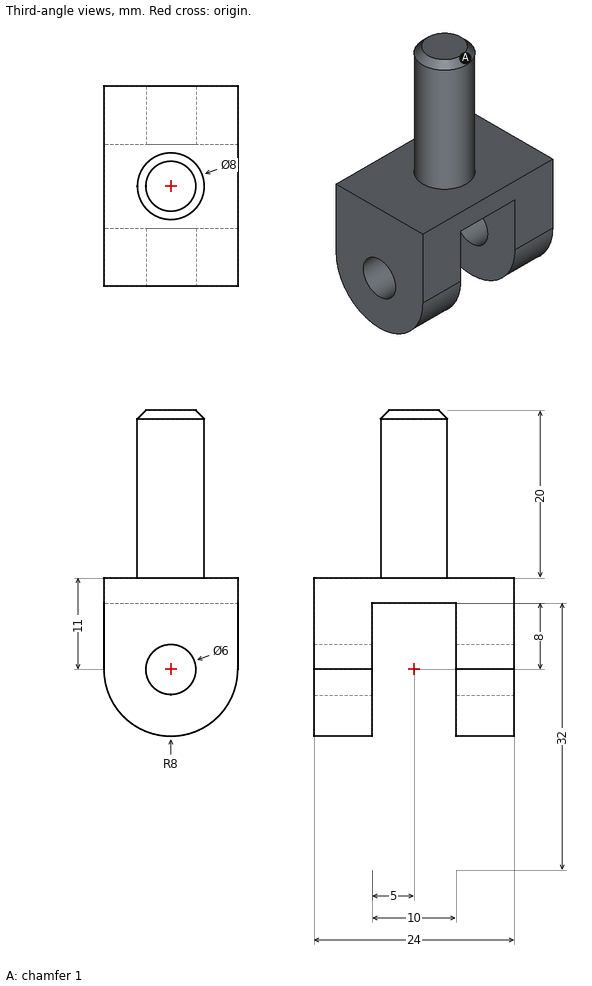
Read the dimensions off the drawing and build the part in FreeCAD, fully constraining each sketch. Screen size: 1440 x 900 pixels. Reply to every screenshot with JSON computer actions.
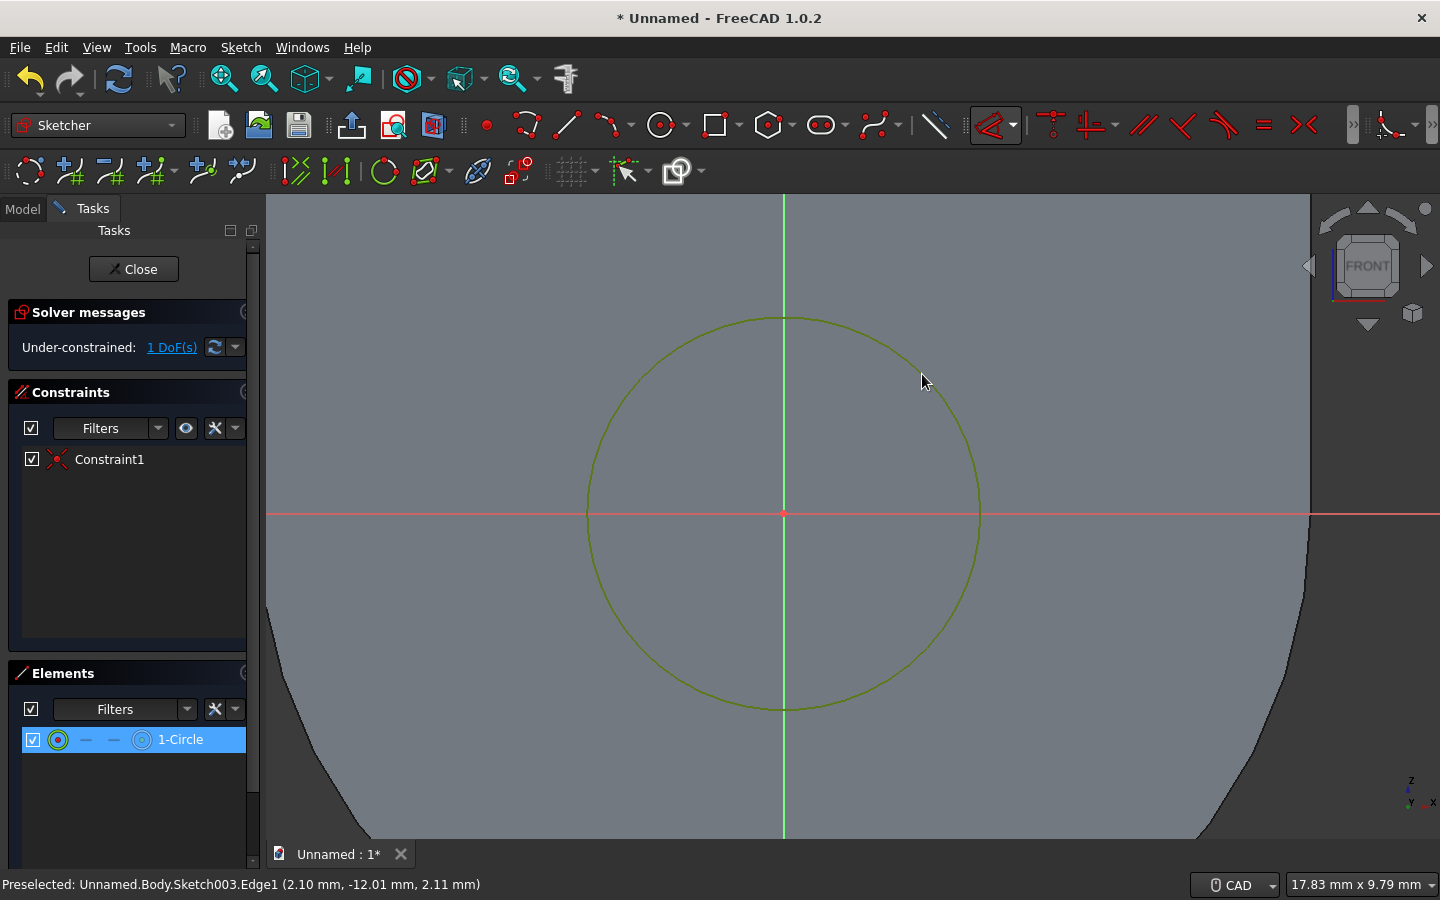
{"action": "left_click", "coordinate": [1016, 126]}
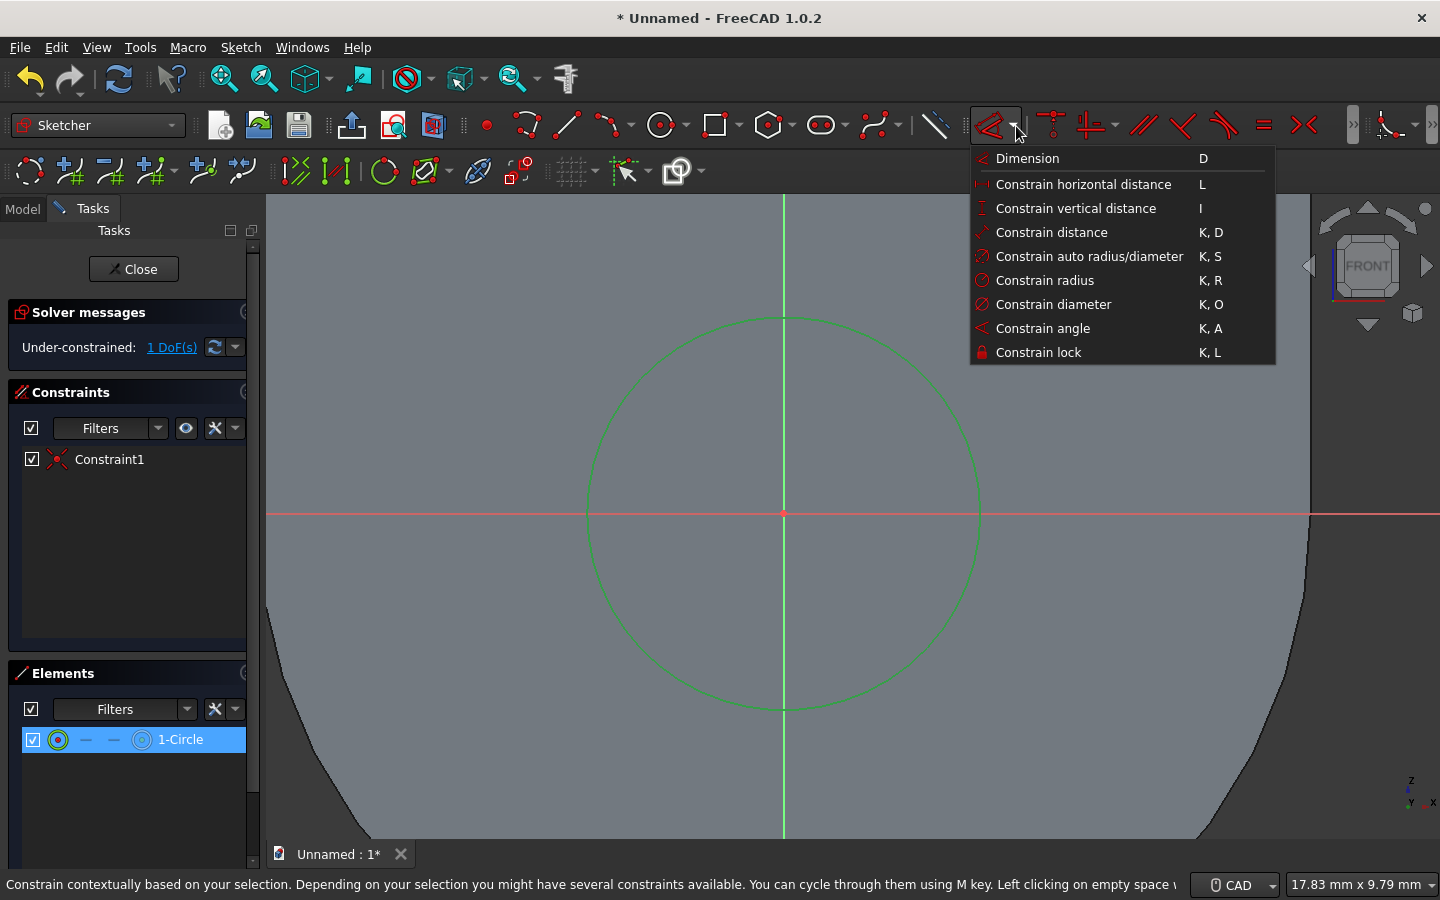
{"action": "left_click", "coordinate": [1123, 304]}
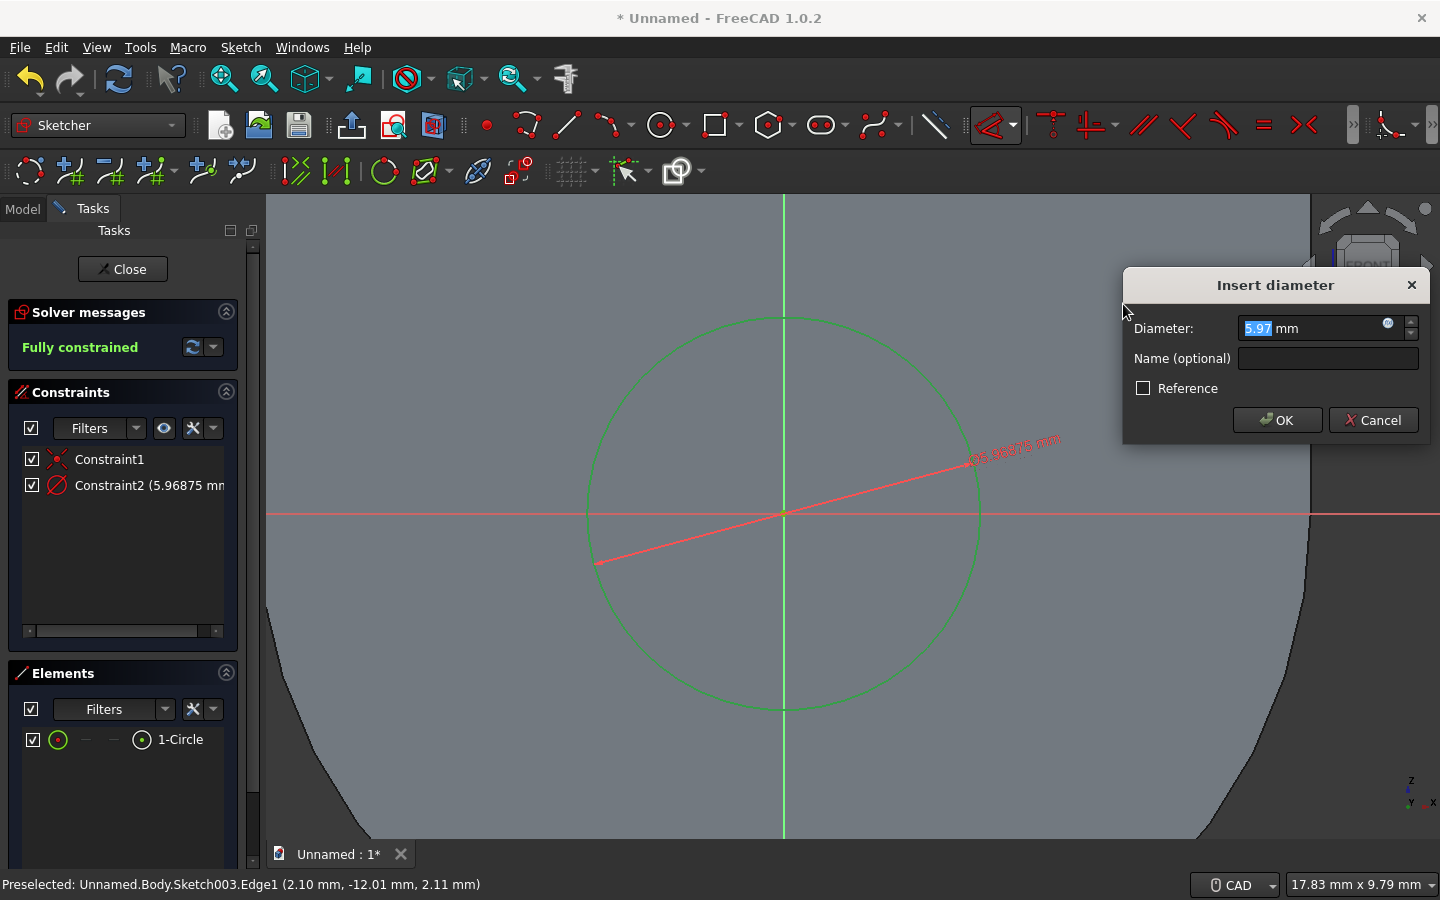
{"action": "type", "text": "6"}
{"action": "key", "text": "Return"}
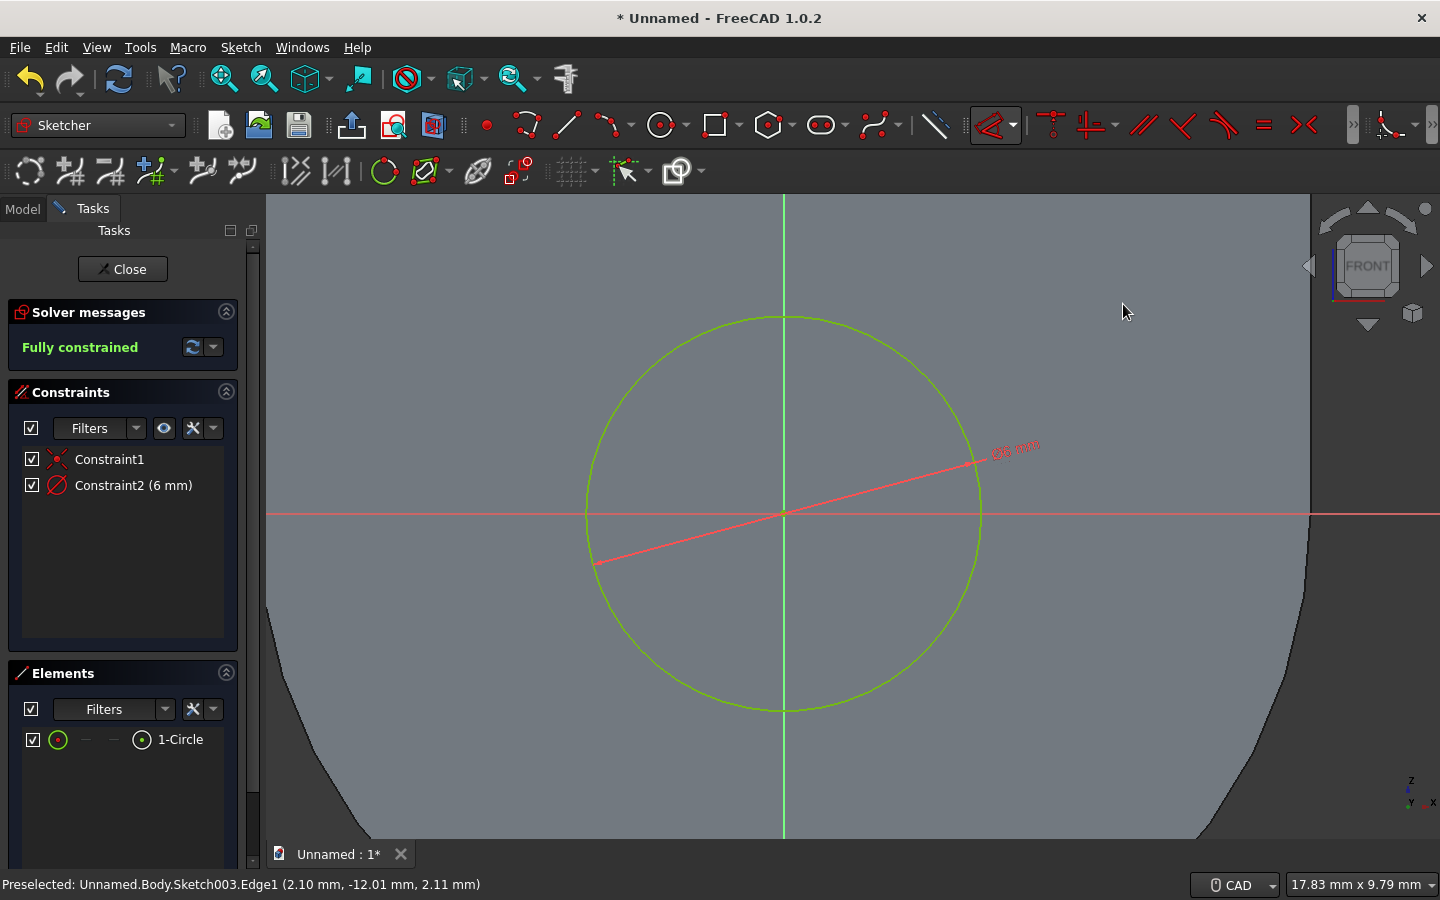
{"action": "left_click", "coordinate": [123, 269]}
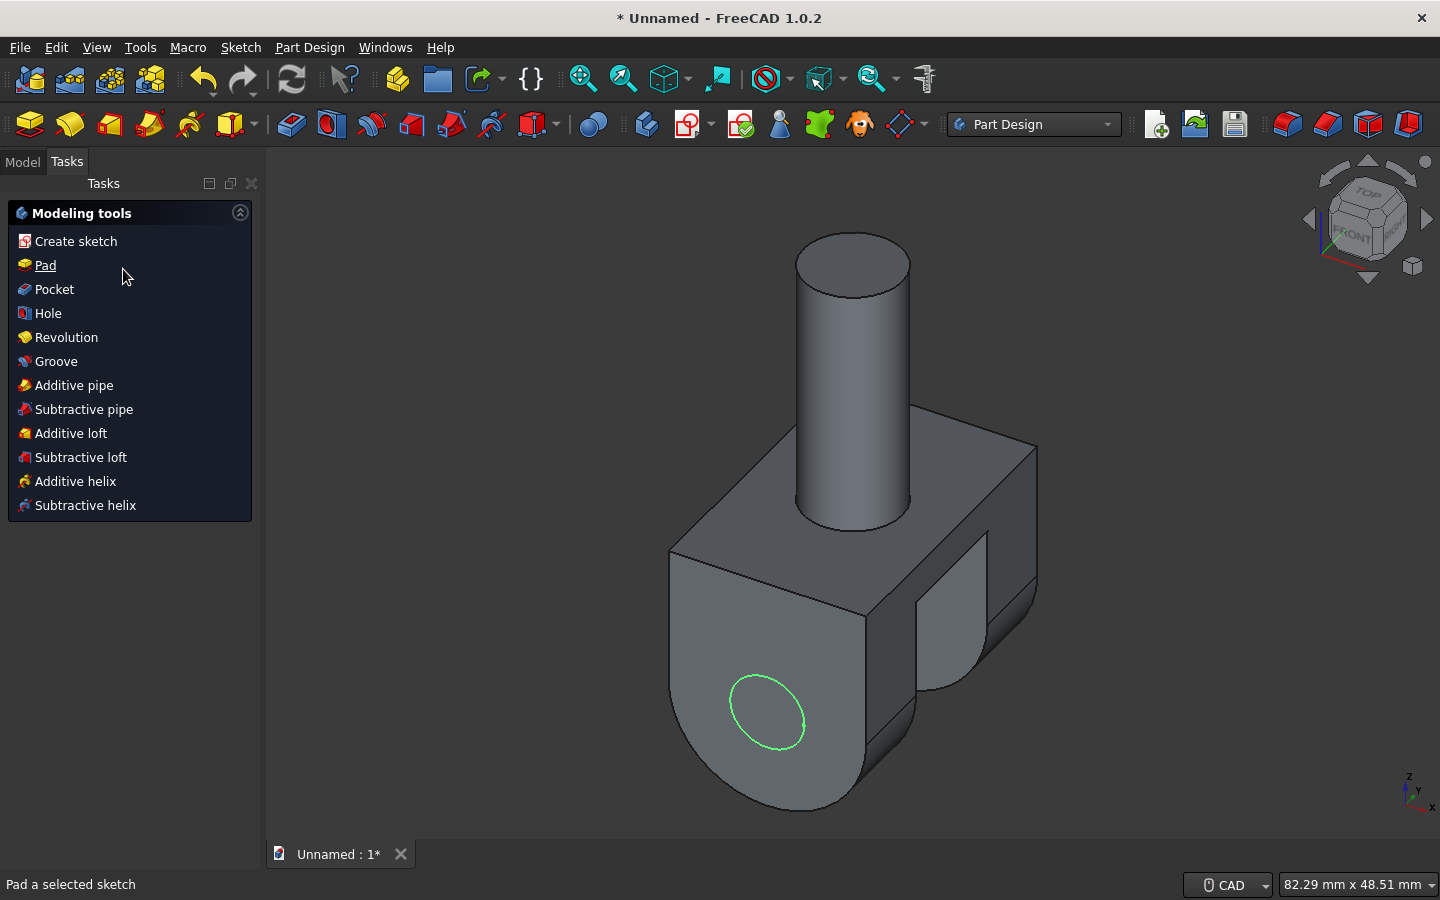
{"action": "left_click", "coordinate": [292, 124]}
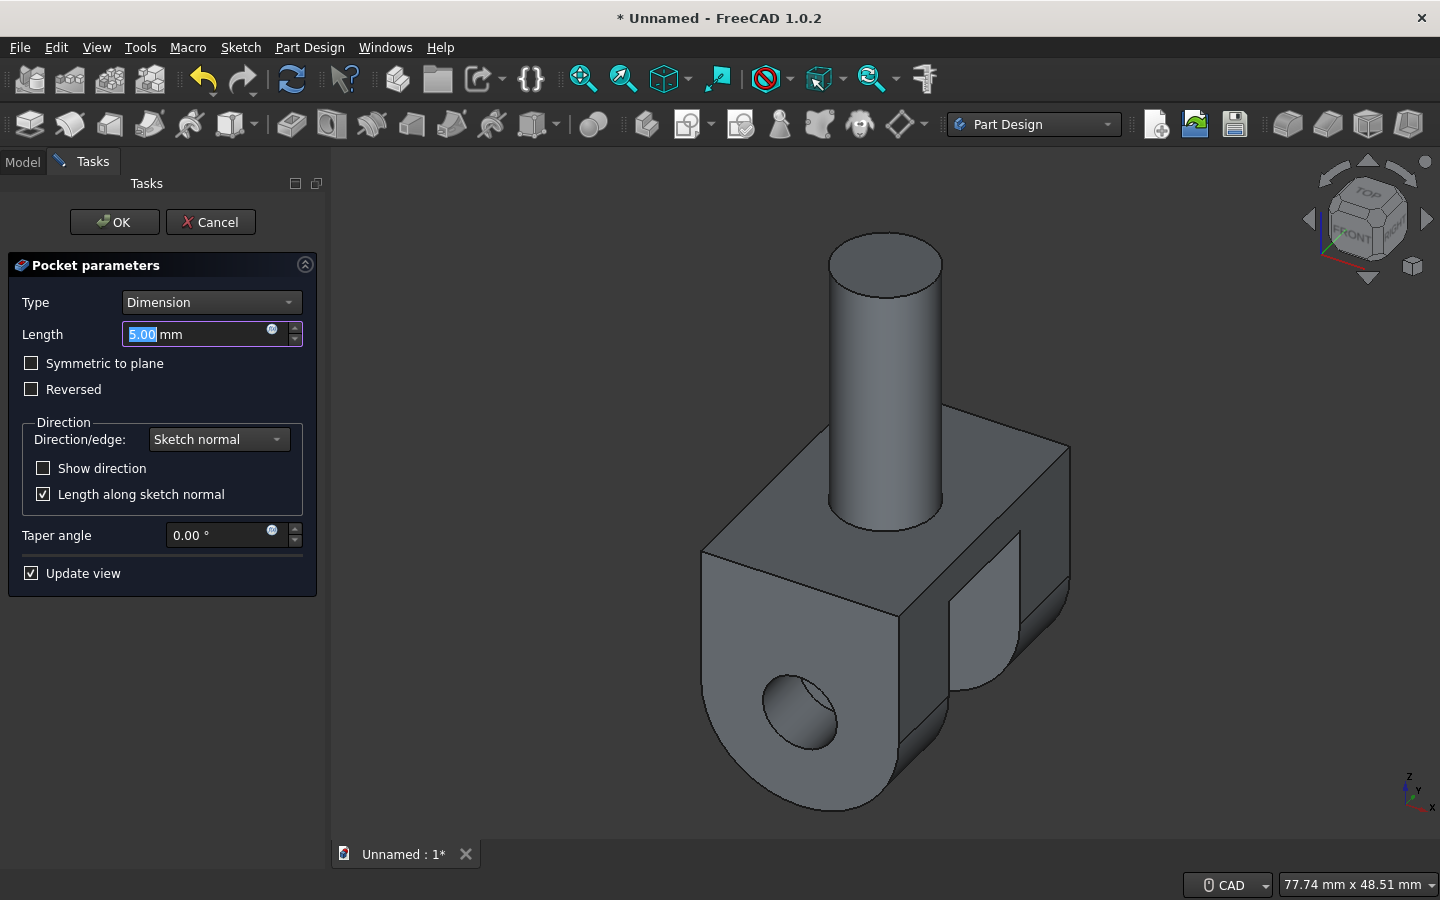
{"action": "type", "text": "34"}
{"action": "key", "text": "Tab"}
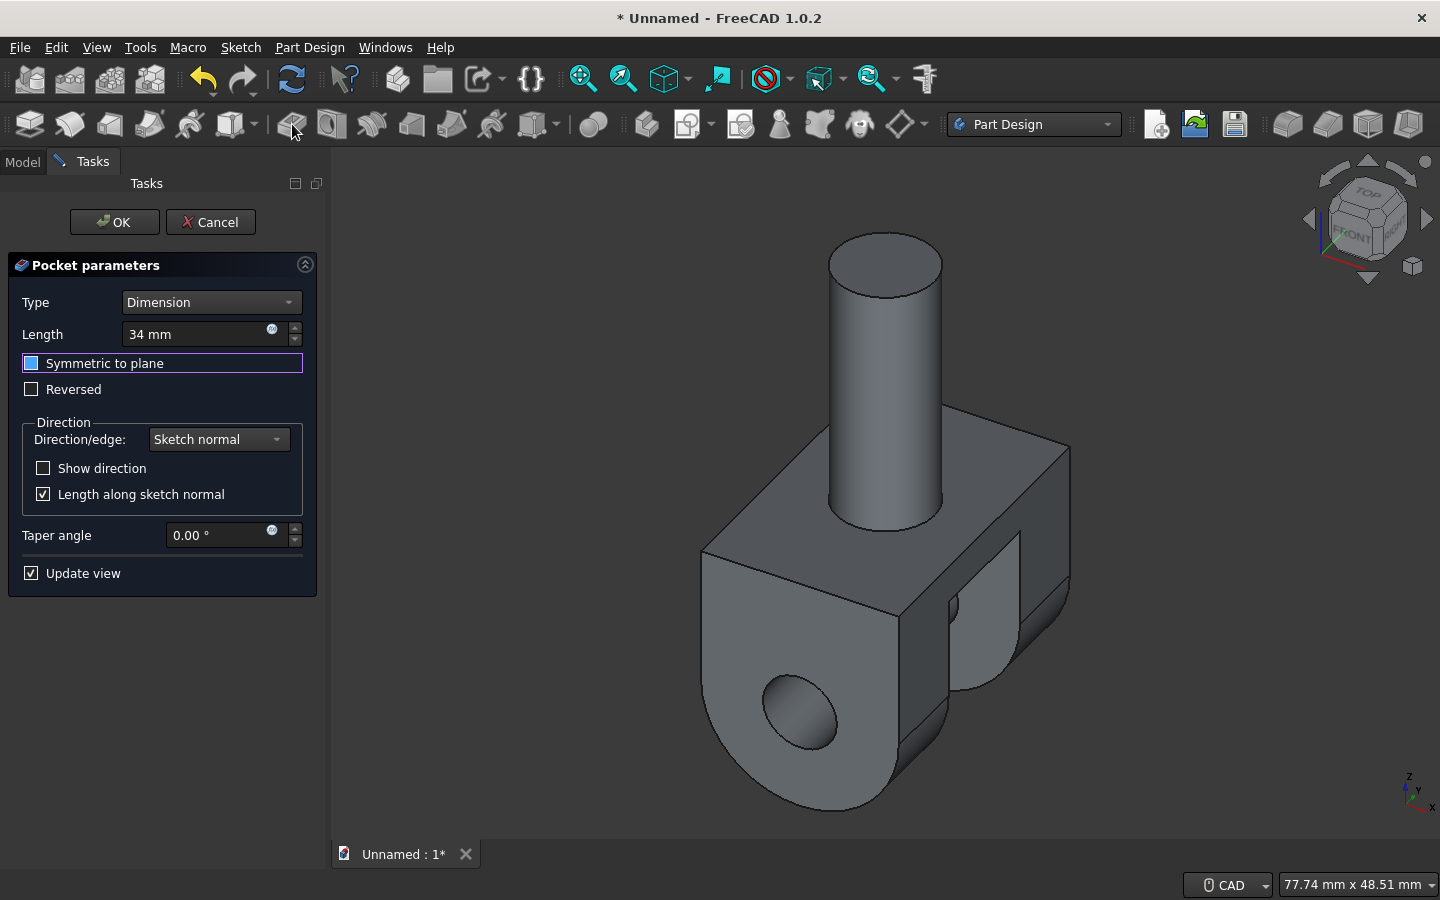
{"action": "left_click", "coordinate": [115, 222]}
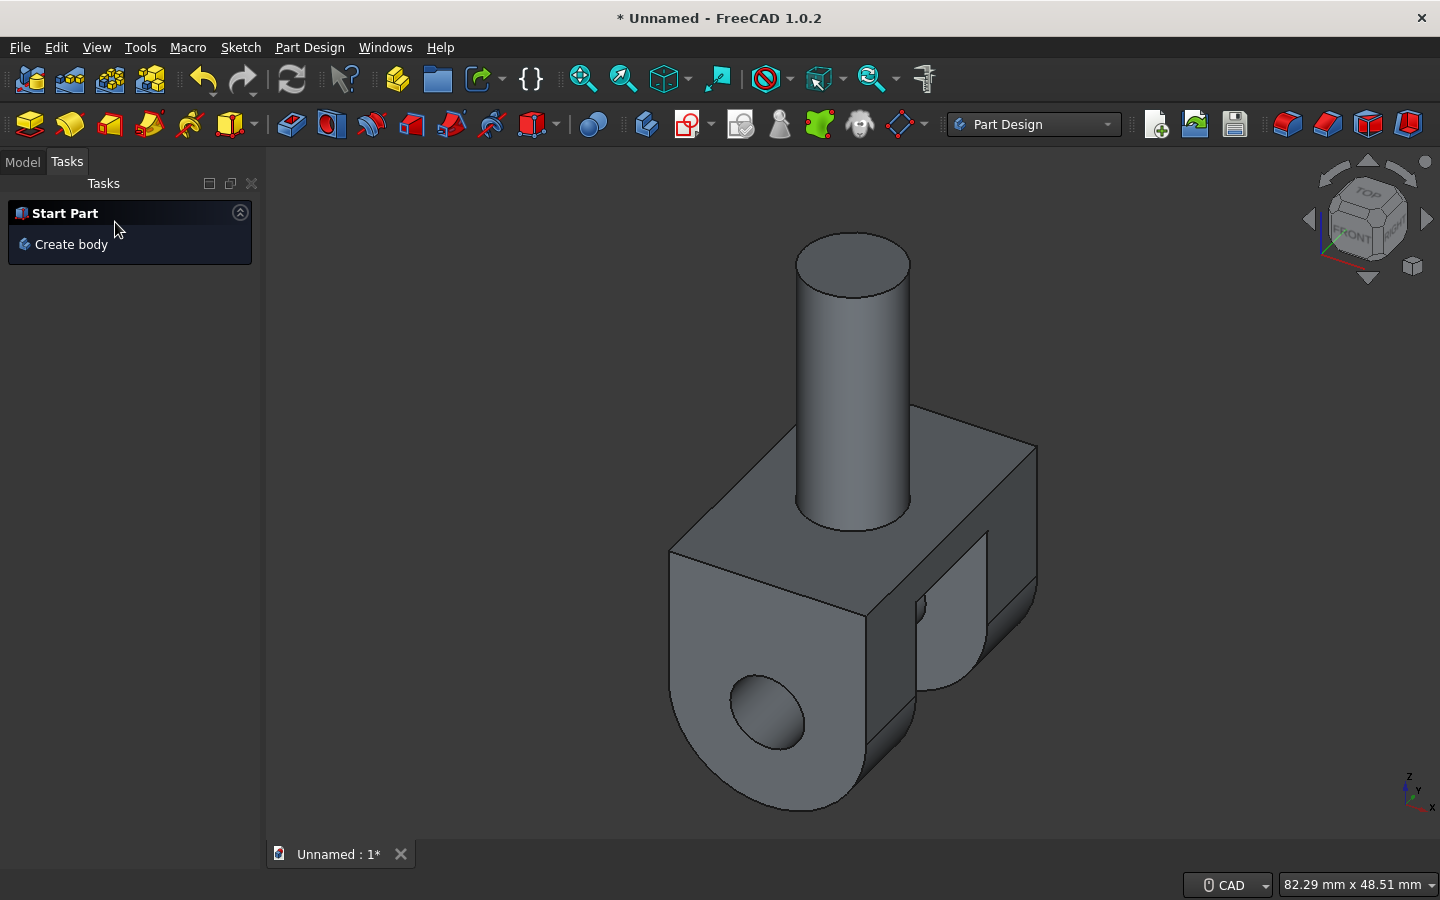
{"action": "left_click", "coordinate": [584, 80]}